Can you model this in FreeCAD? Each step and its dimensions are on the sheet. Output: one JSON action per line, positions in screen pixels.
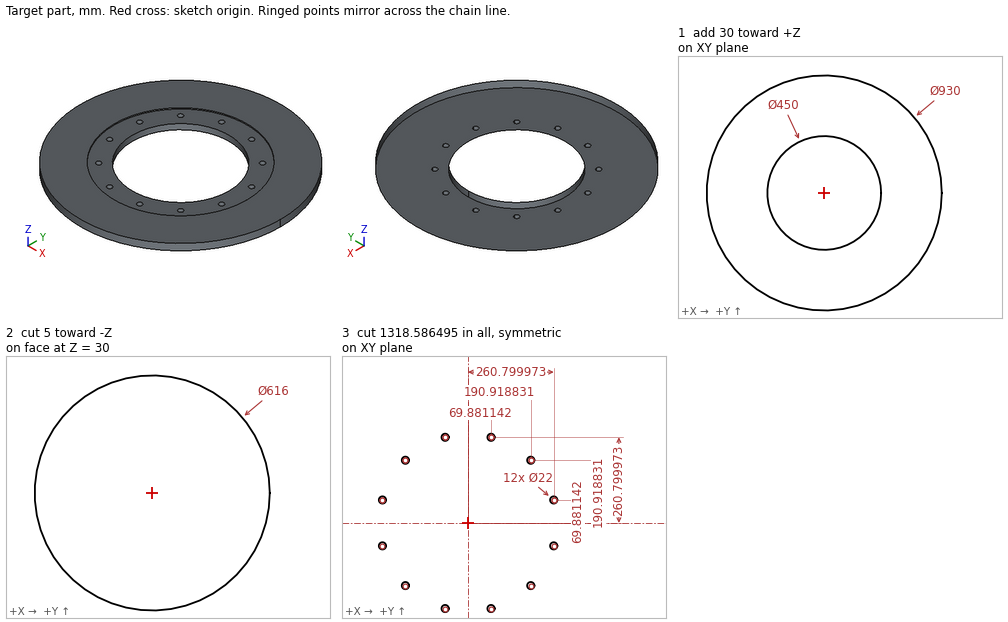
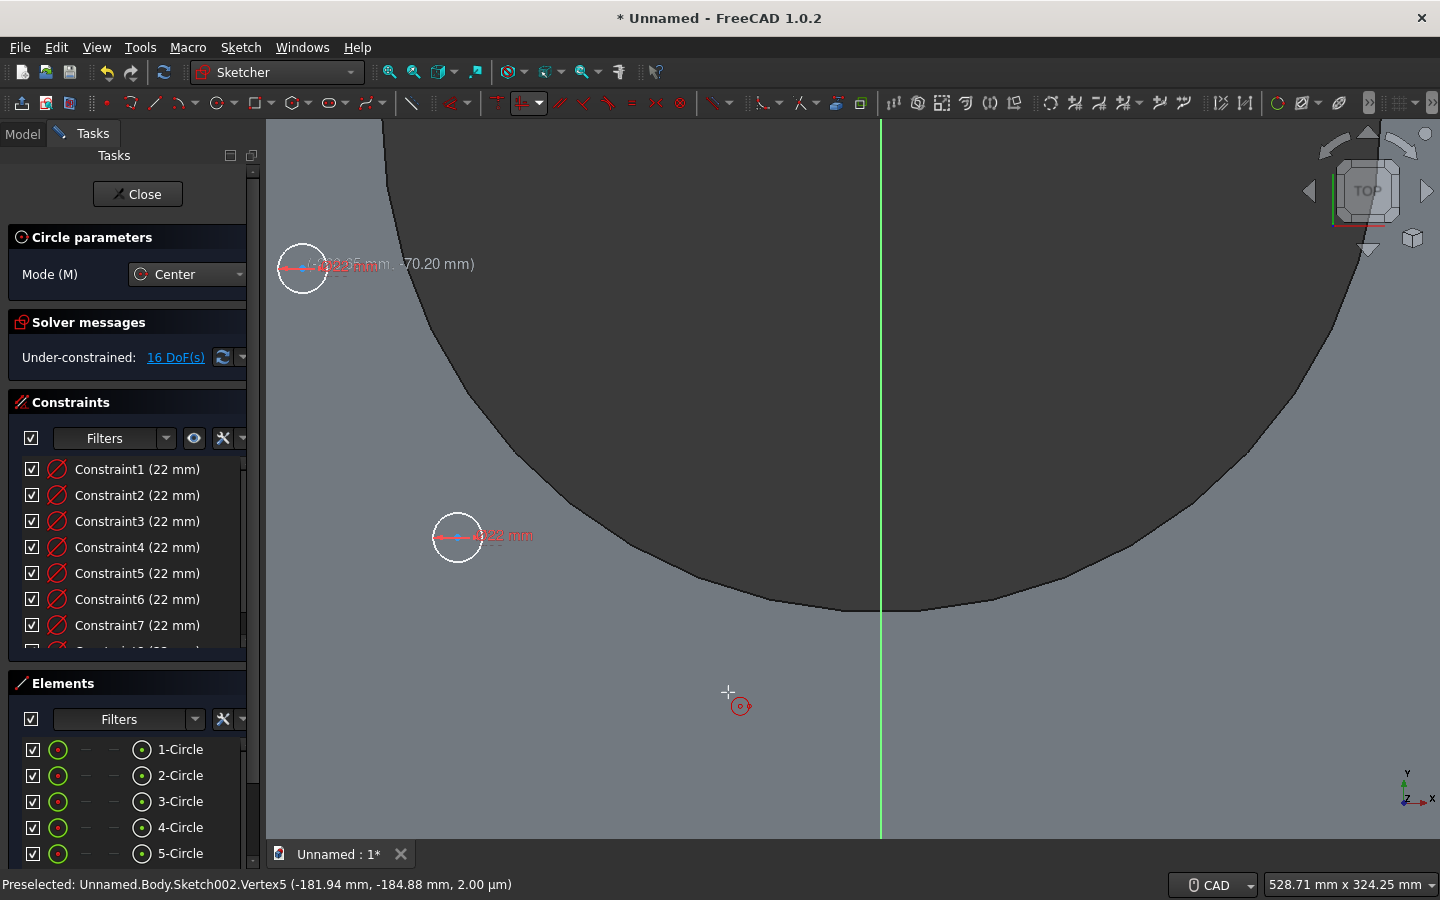
{"action": "left_click", "coordinate": [726, 692]}
{"action": "mouse_move", "coordinate": [744, 675]}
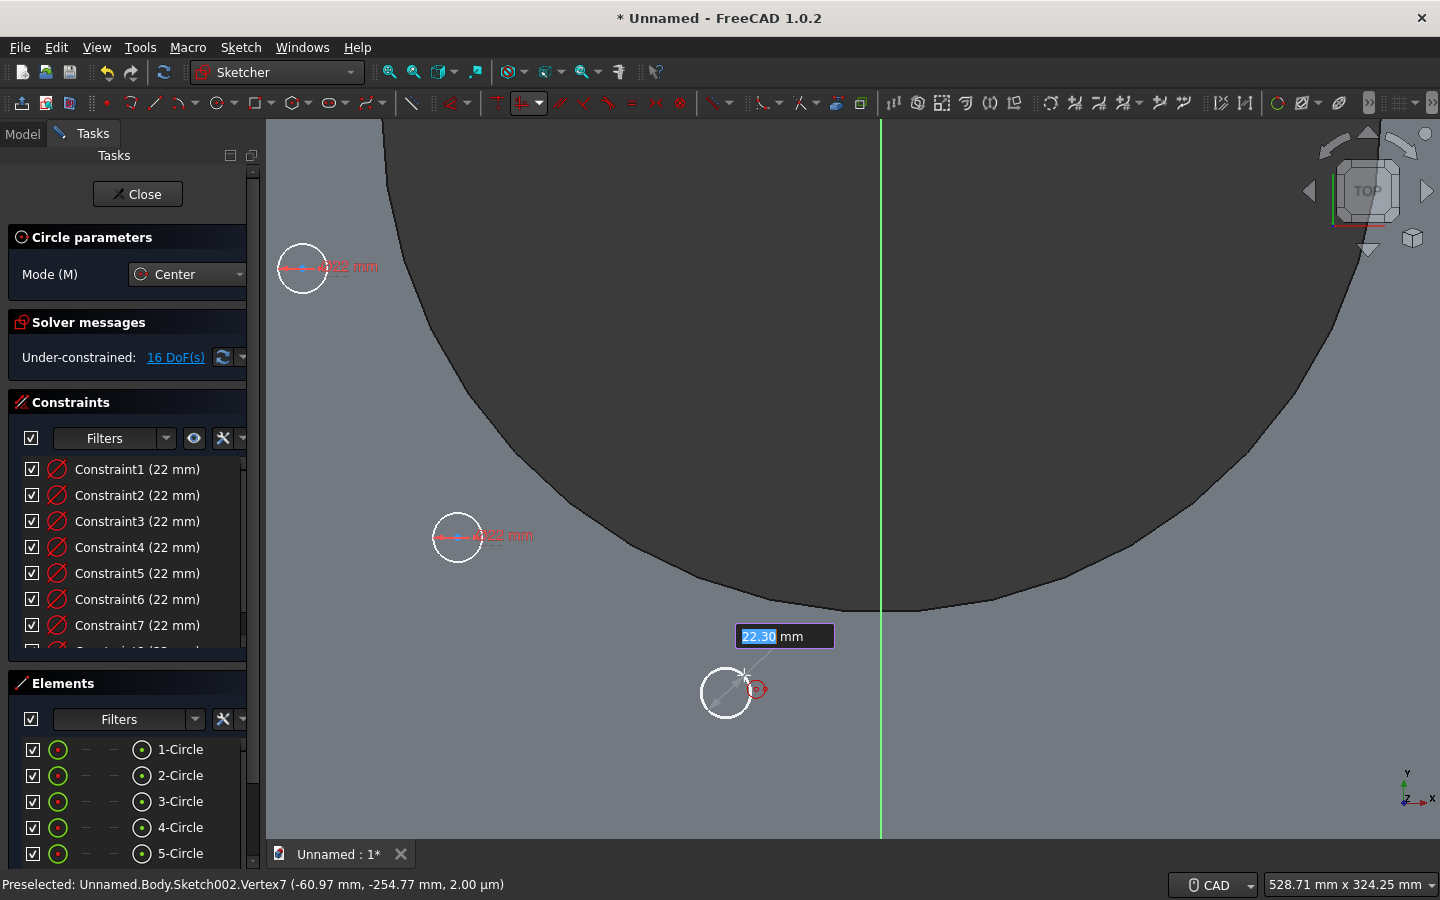
{"action": "type", "text": "22"}
{"action": "key", "text": "Return"}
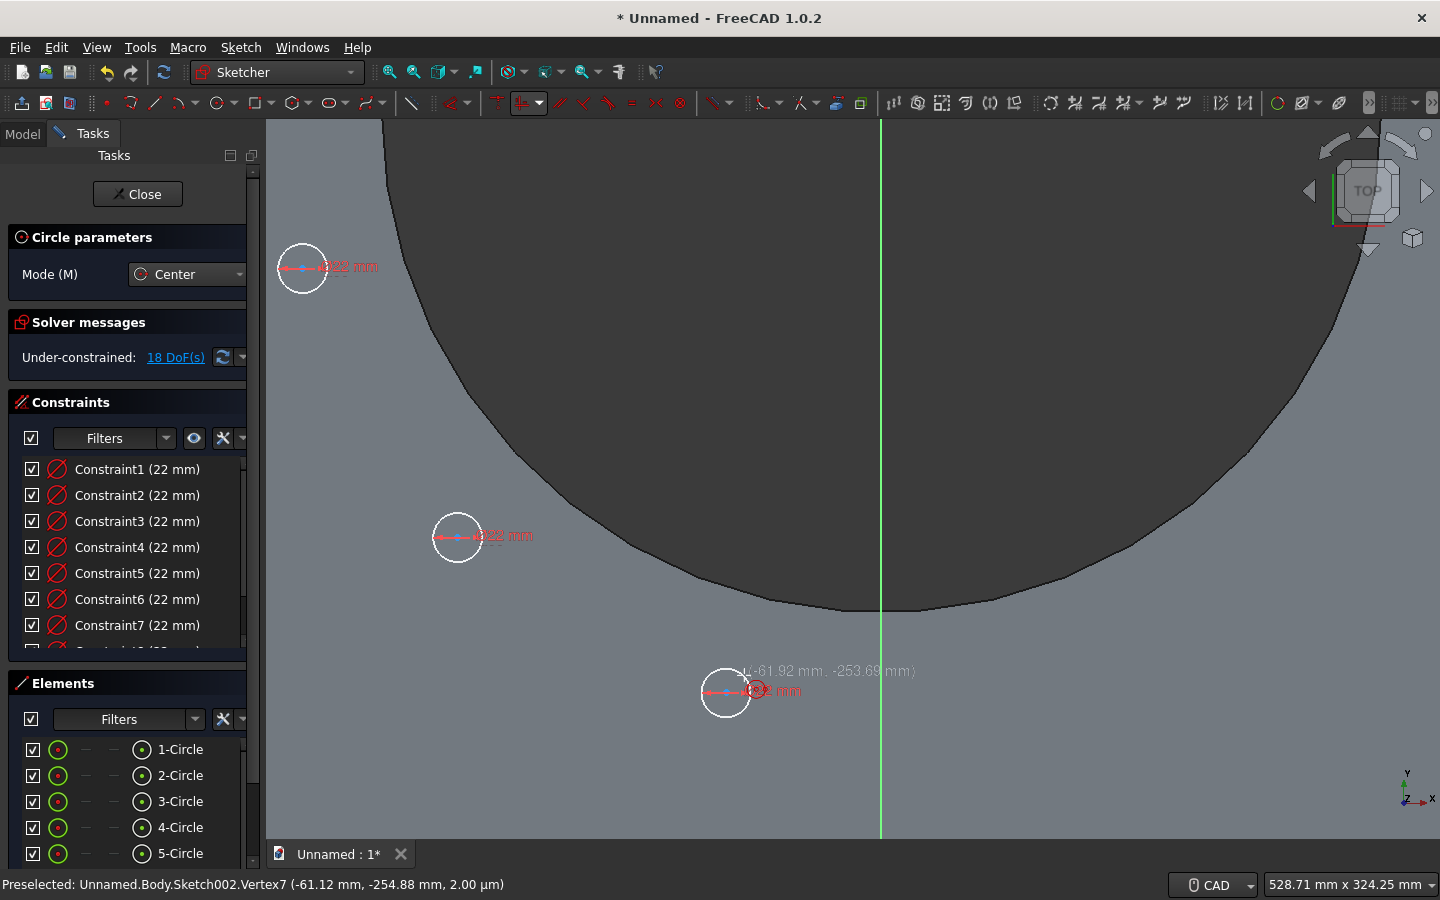
{"action": "left_click", "coordinate": [1037, 692]}
{"action": "mouse_move", "coordinate": [1054, 675]}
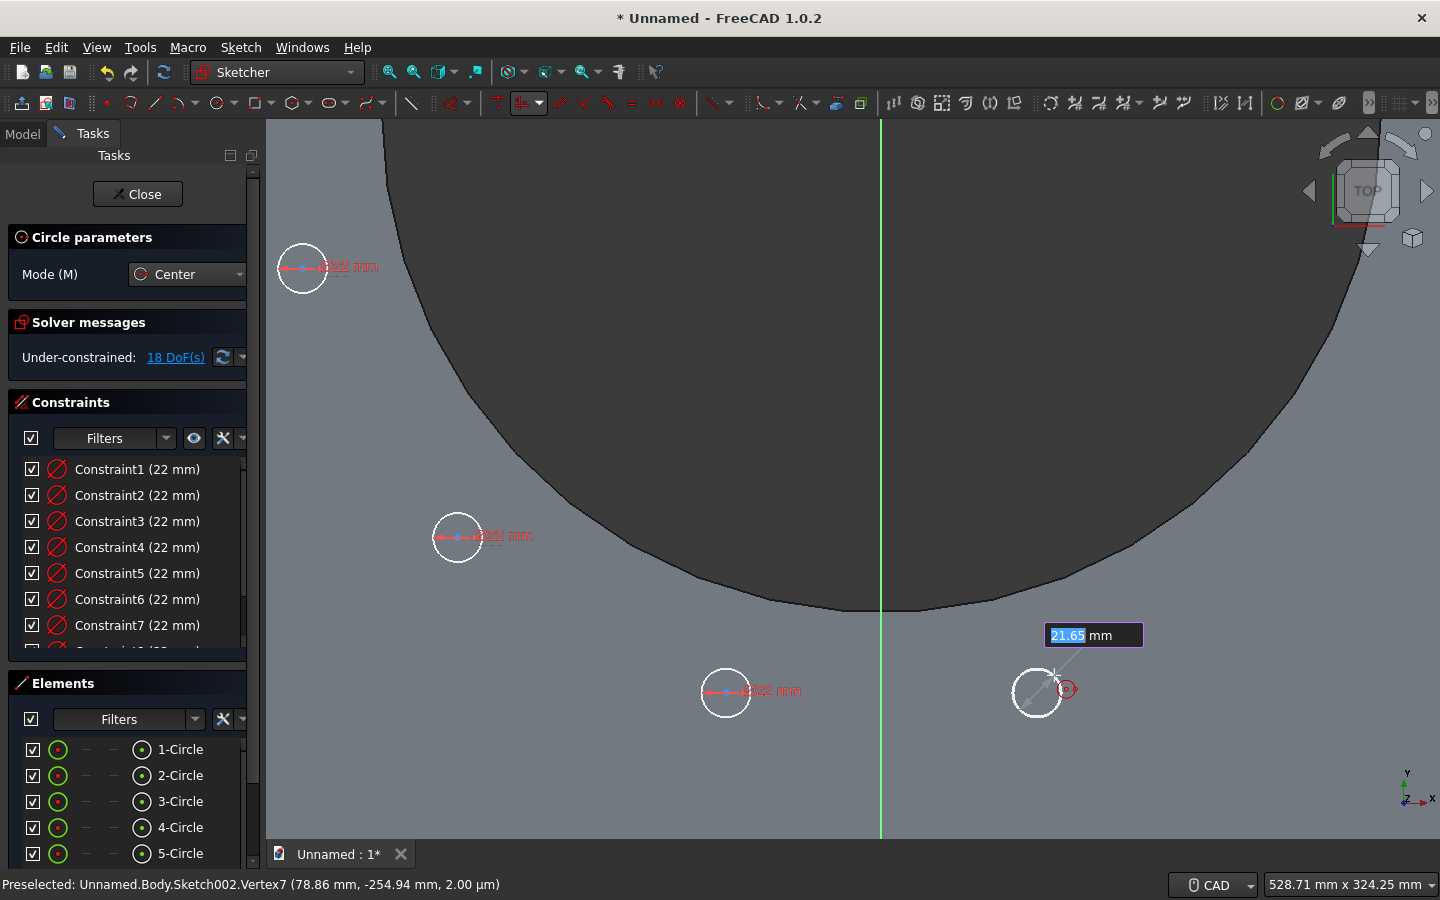
{"action": "type", "text": "22"}
{"action": "key", "text": "Return"}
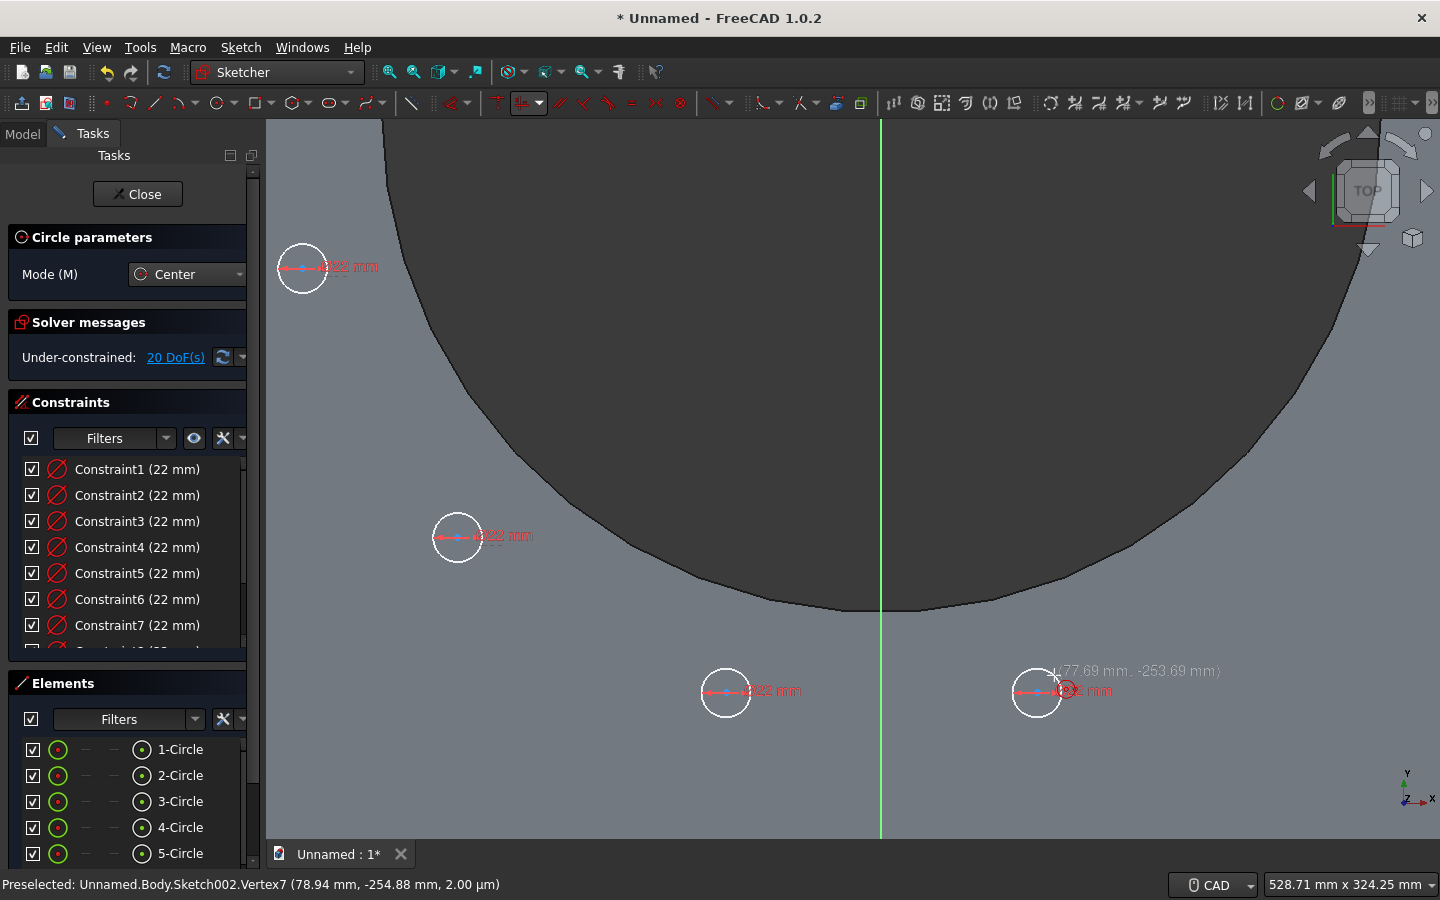
{"action": "scroll", "coordinate": [728, 692], "scroll_direction": "down", "scroll_amount": 5}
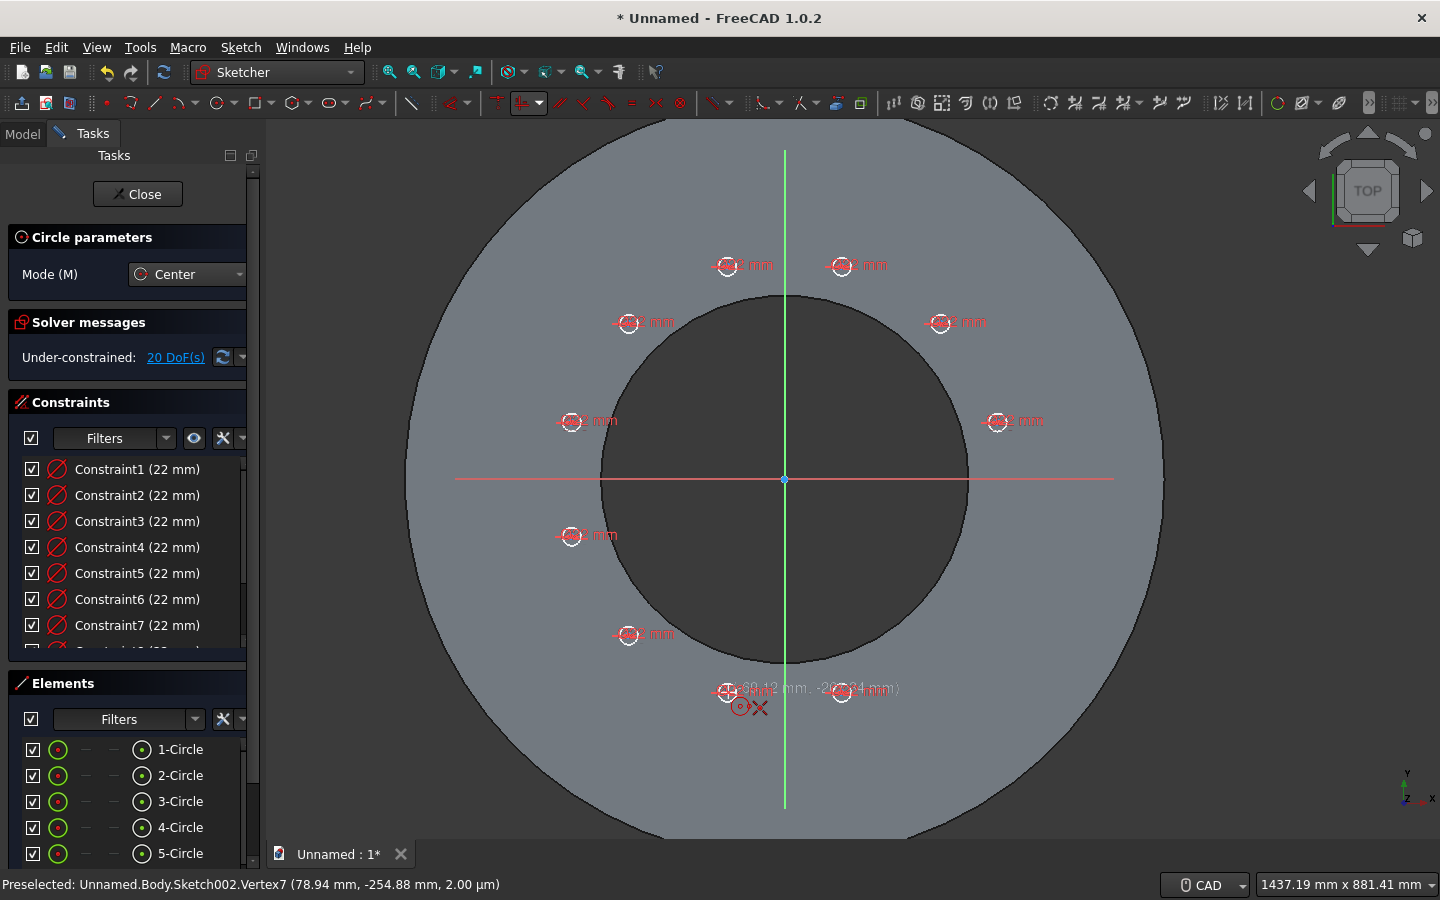
{"action": "scroll", "coordinate": [941, 635], "scroll_direction": "up", "scroll_amount": 5}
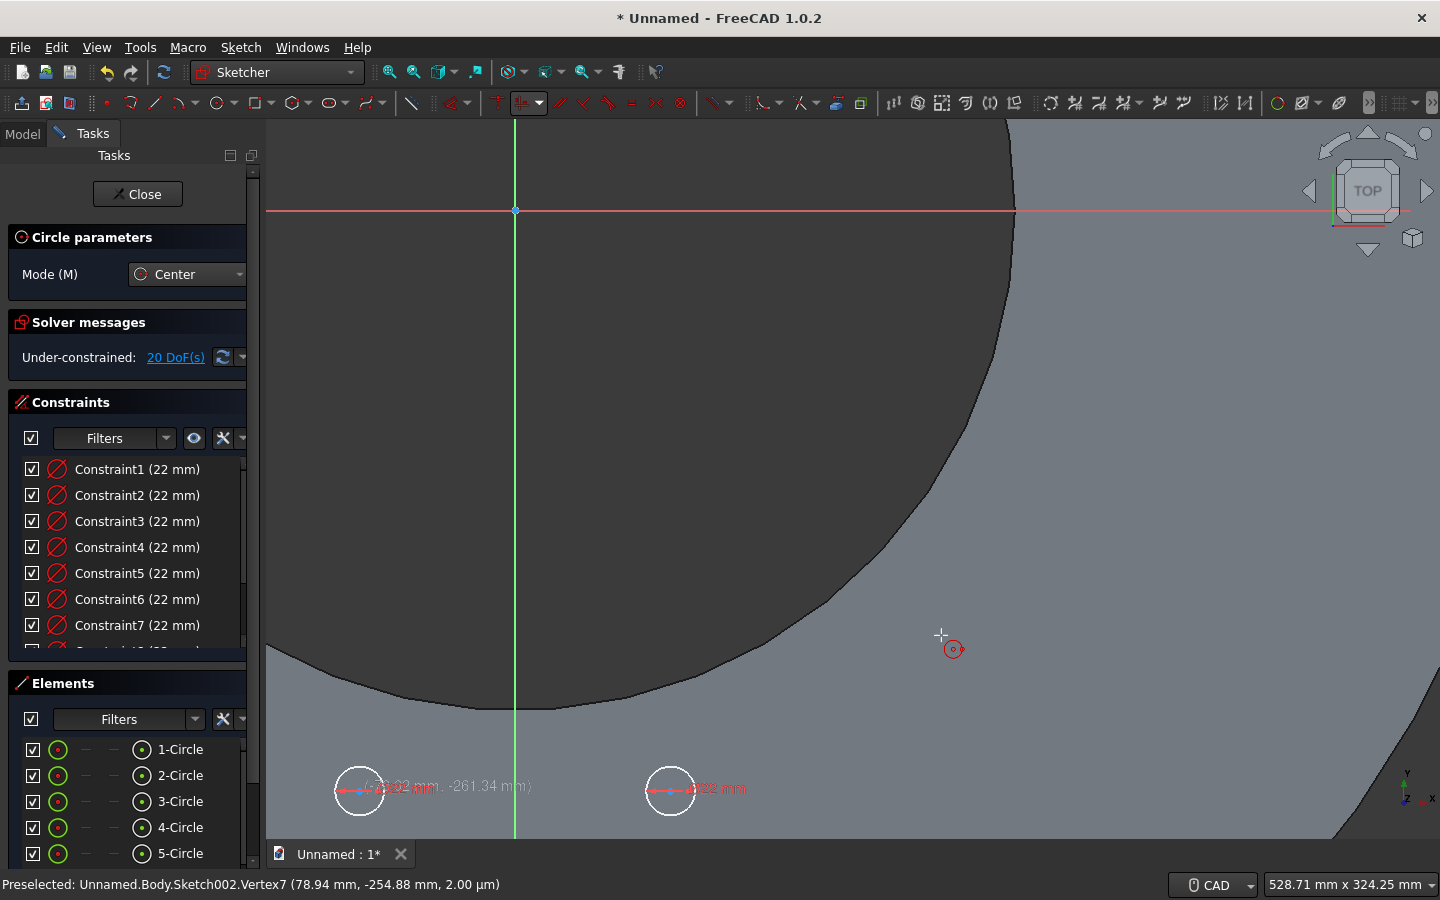
{"action": "left_click", "coordinate": [939, 635]}
{"action": "mouse_move", "coordinate": [956, 617]}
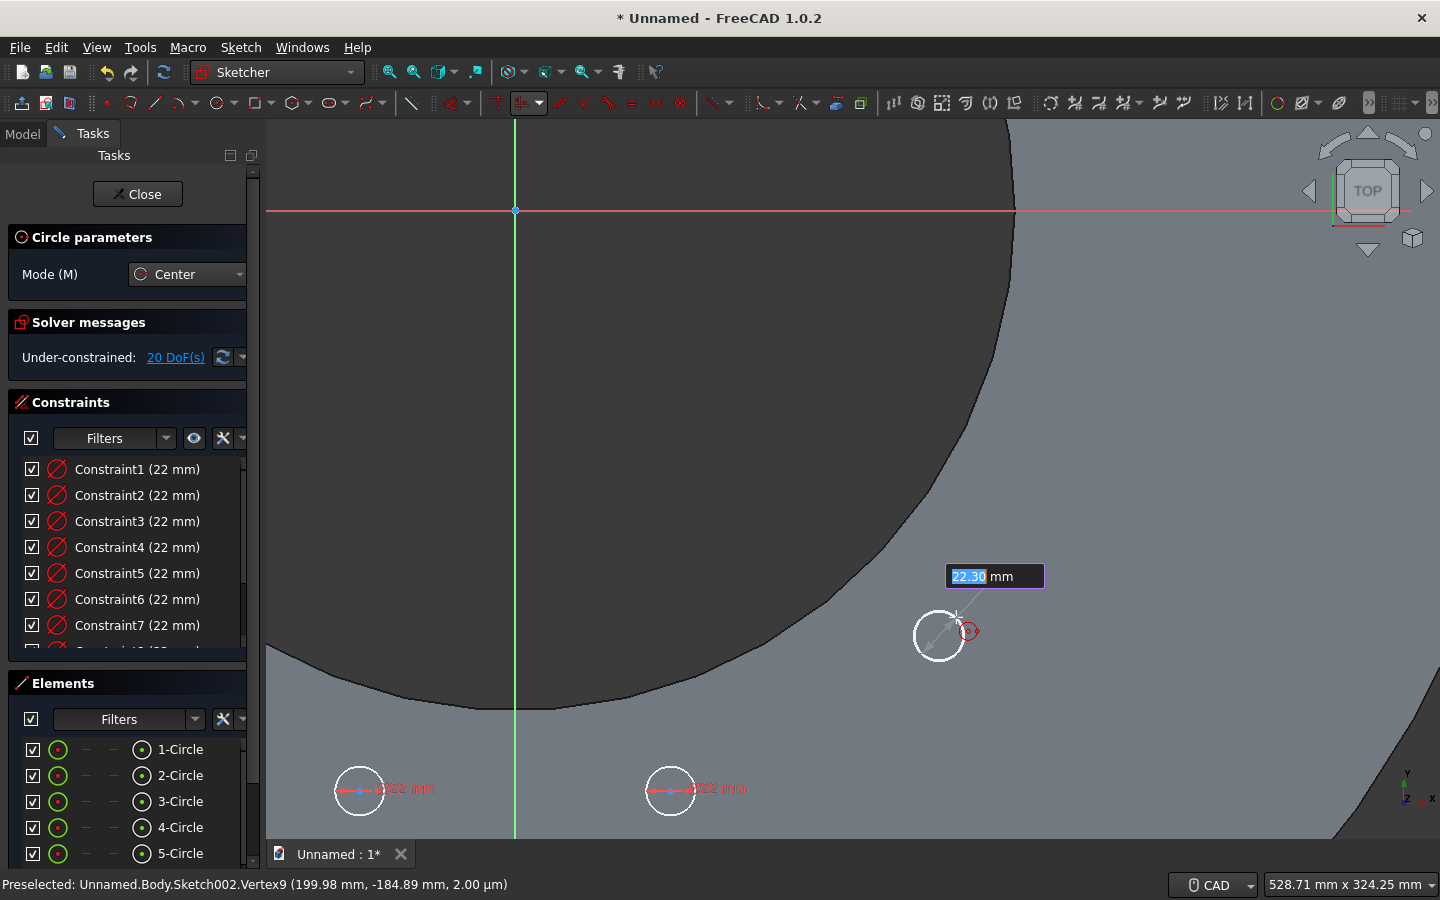
{"action": "type", "text": "22"}
{"action": "key", "text": "Return"}